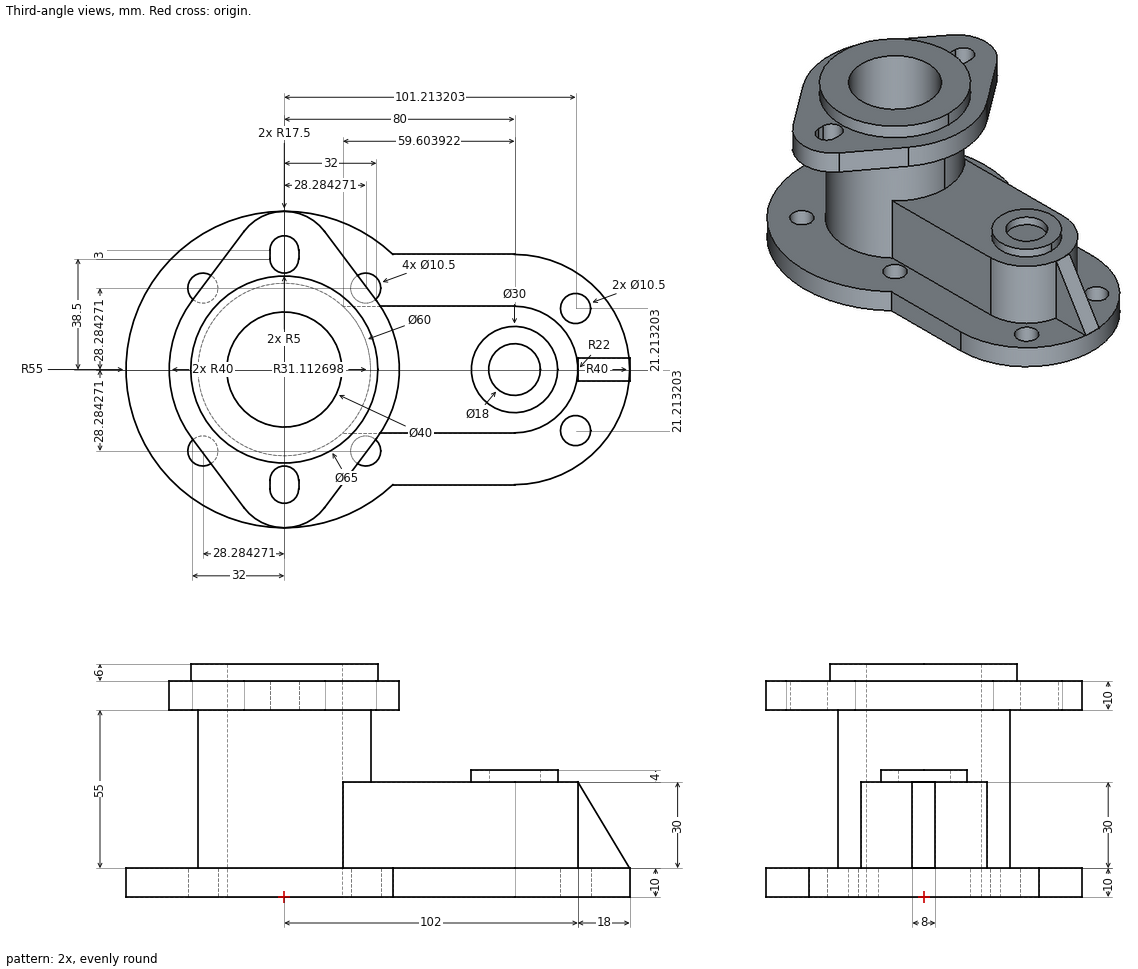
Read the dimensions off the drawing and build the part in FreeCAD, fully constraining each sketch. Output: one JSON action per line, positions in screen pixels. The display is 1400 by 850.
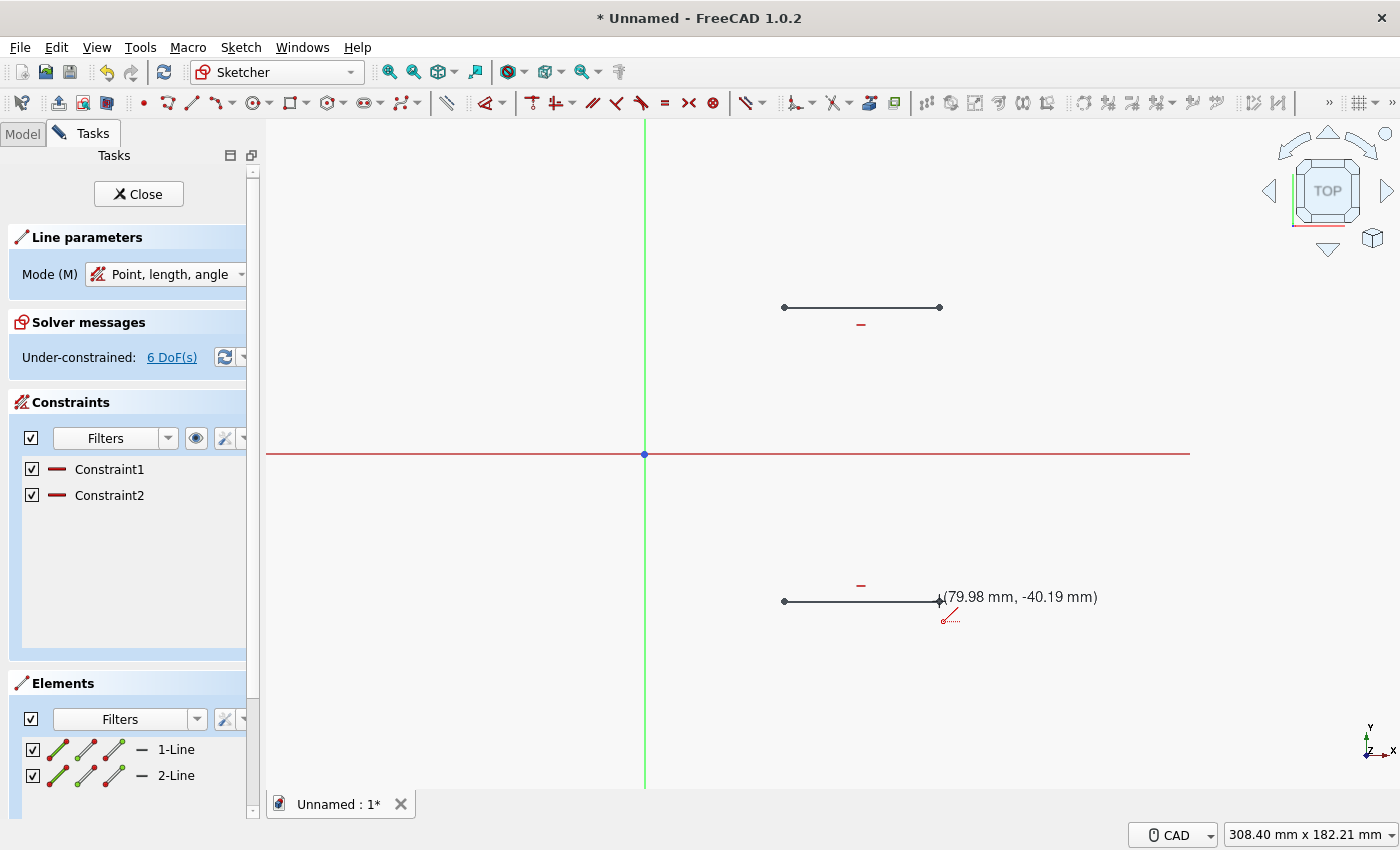
{"action": "key", "text": "g 3 a"}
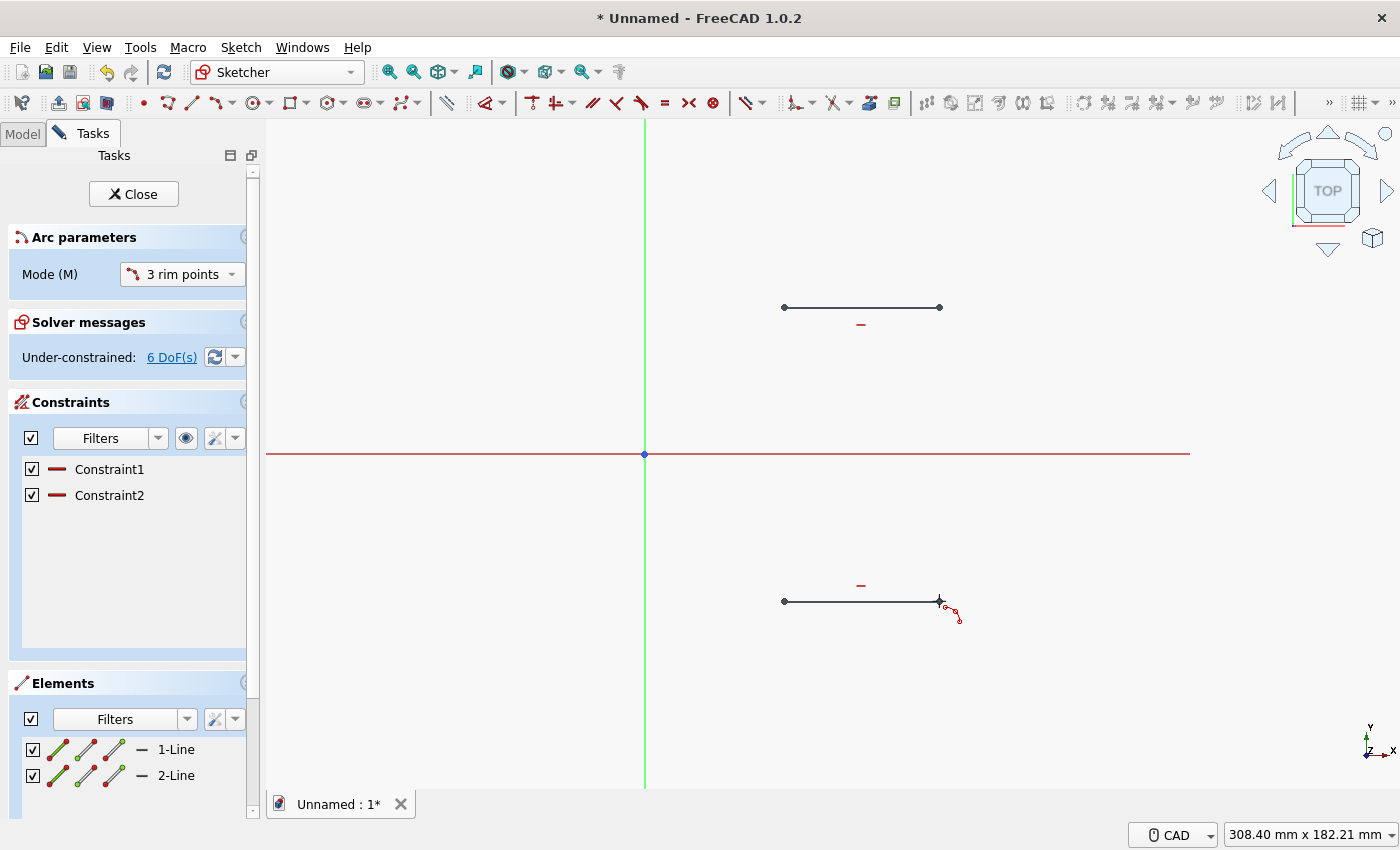
{"action": "left_click", "coordinate": [784, 308]}
{"action": "left_click", "coordinate": [784, 602]}
{"action": "left_click", "coordinate": [464, 363]}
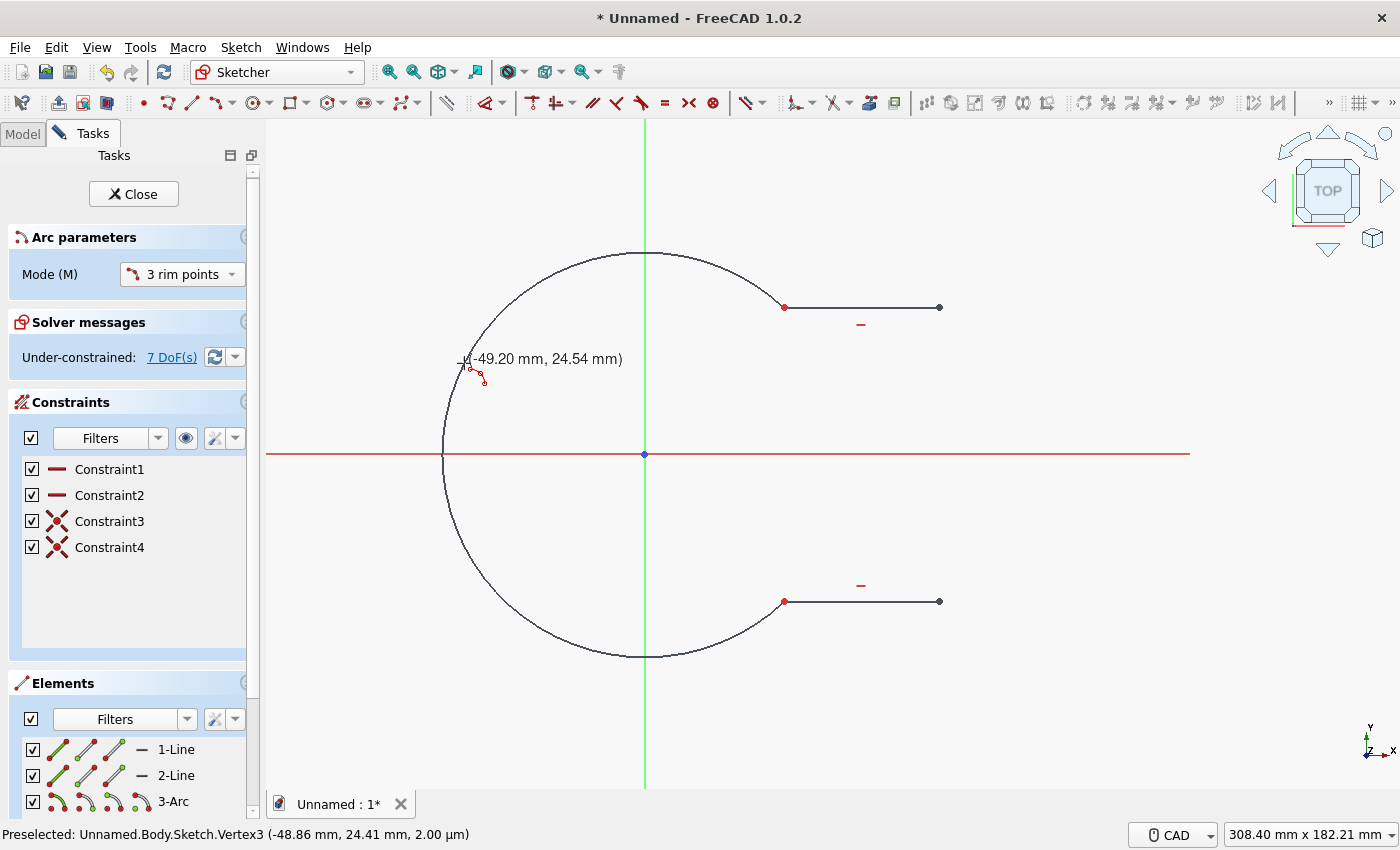
{"action": "left_click", "coordinate": [939, 602]}
{"action": "left_click", "coordinate": [939, 308]}
{"action": "left_click", "coordinate": [1079, 500]}
{"action": "key", "text": "Escape"}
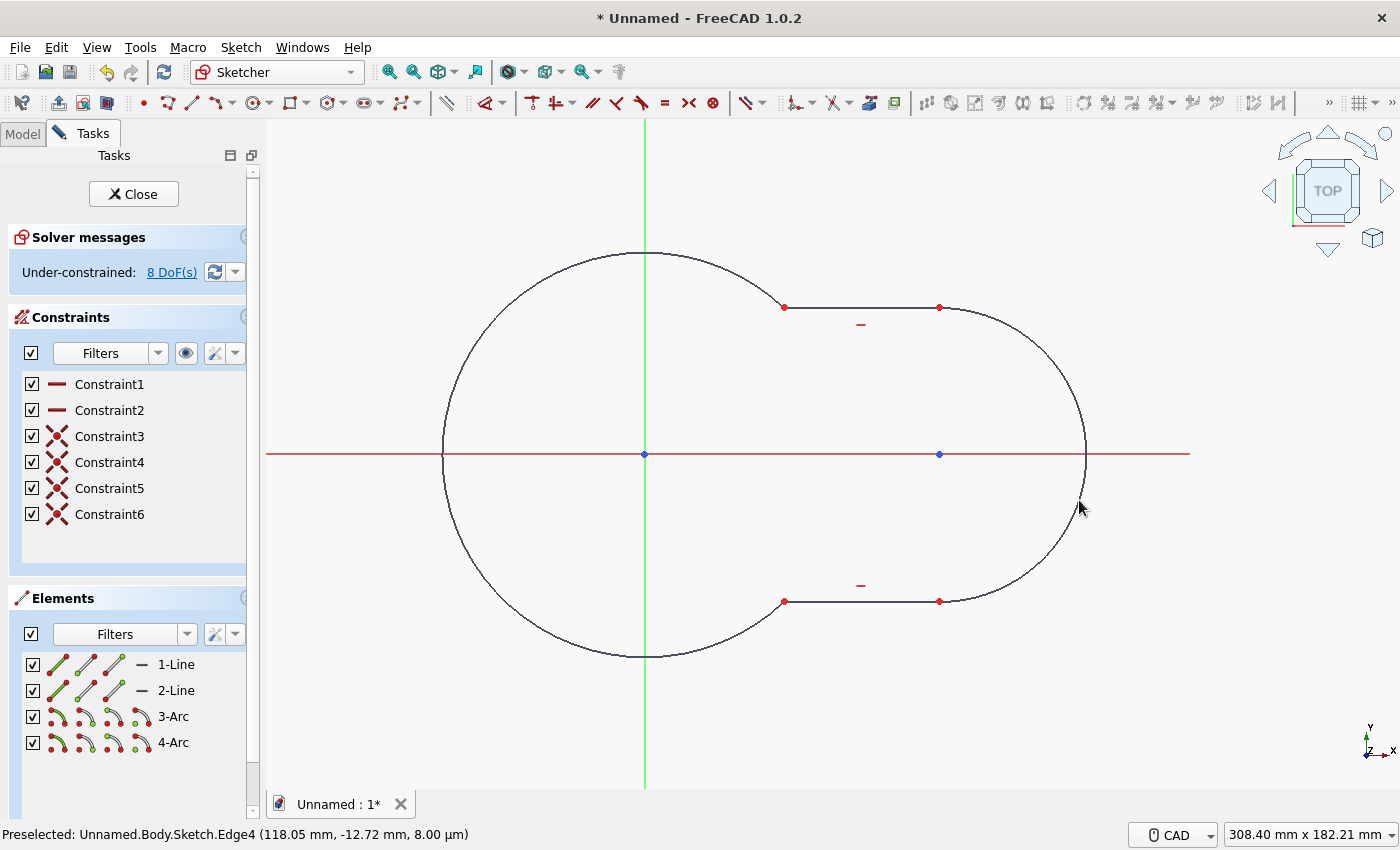
{"action": "left_click_drag", "start_coordinate": [635, 444], "coordinate": [655, 465]}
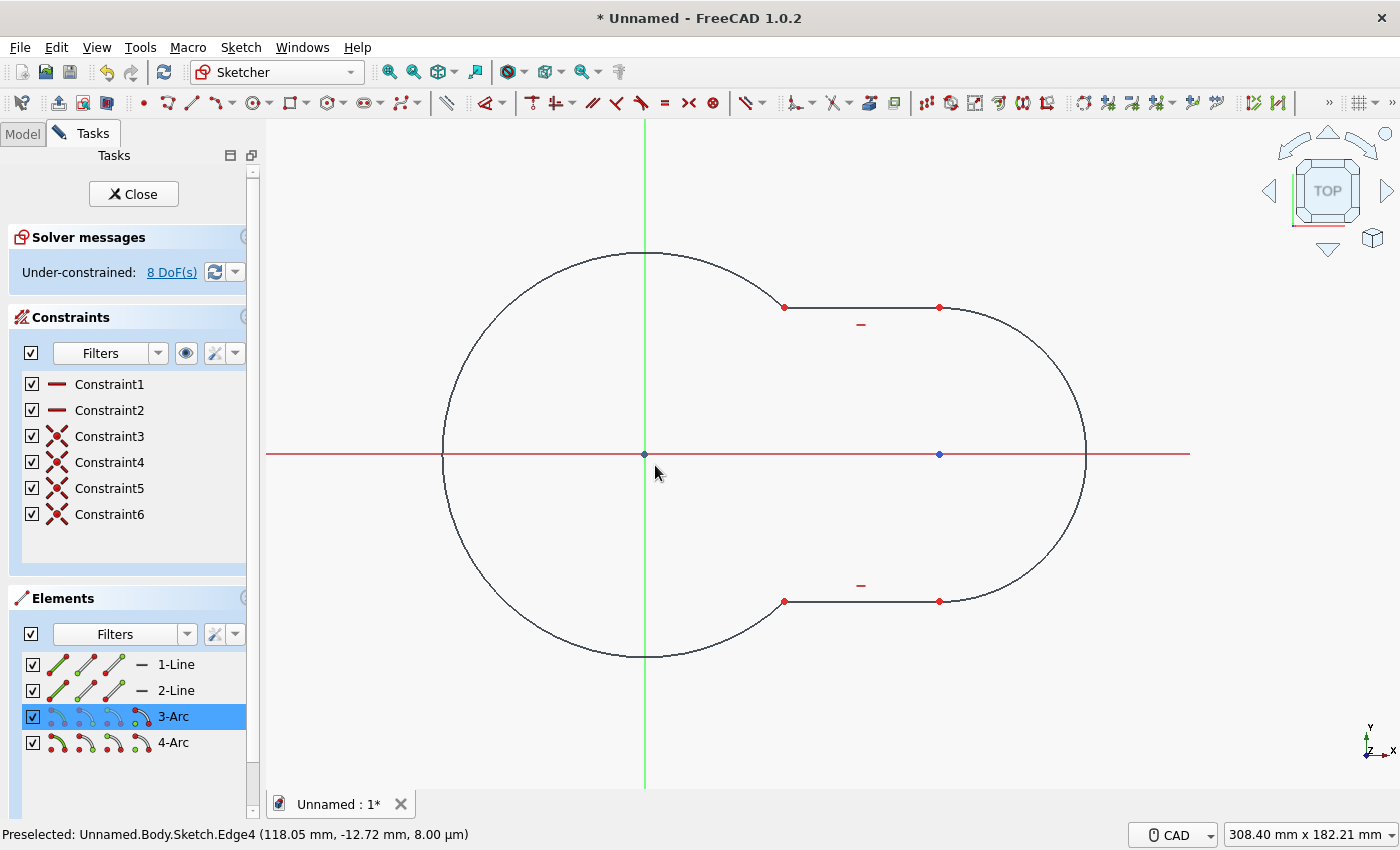
{"action": "key", "text": "c"}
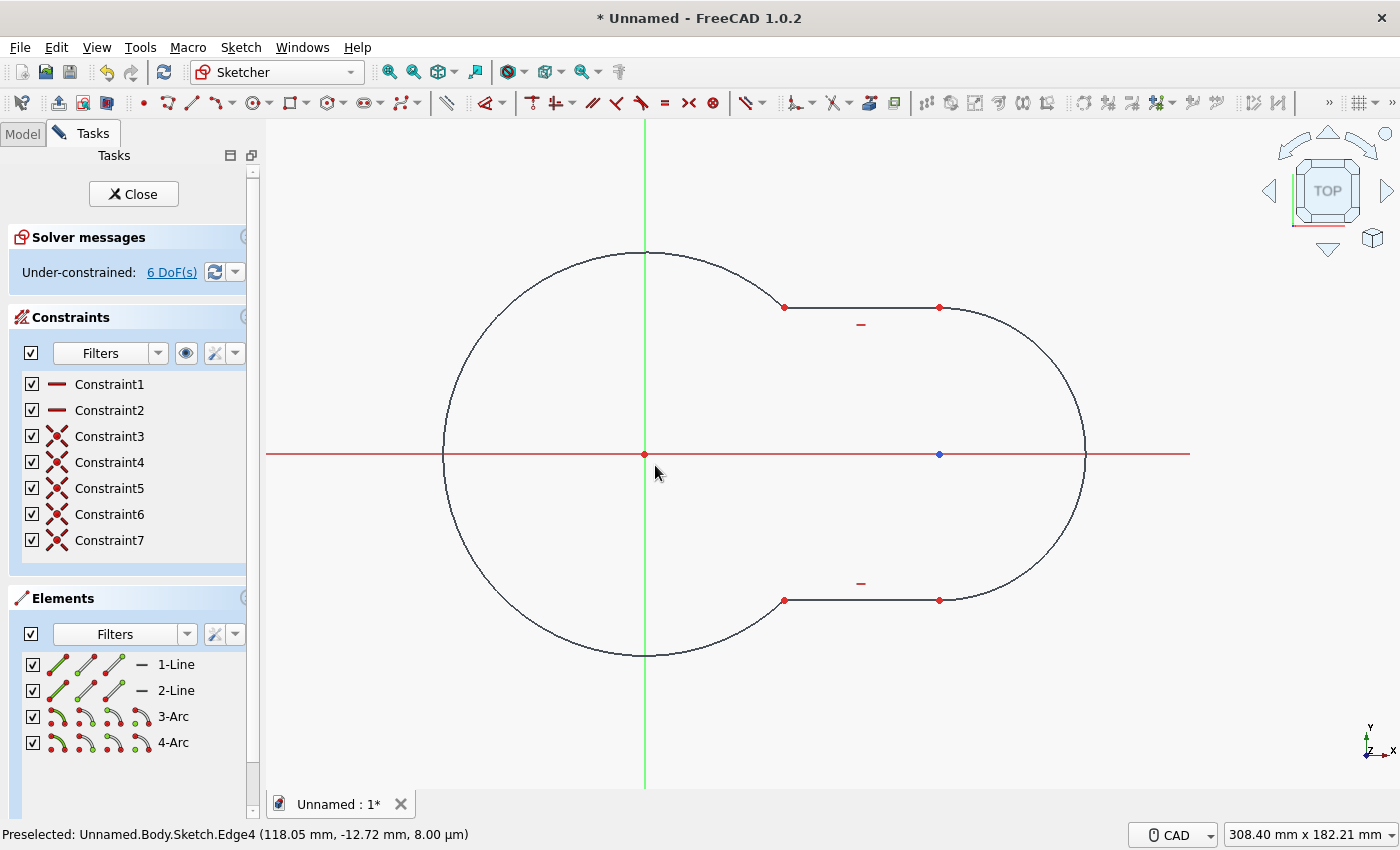
{"action": "left_click", "coordinate": [939, 454]}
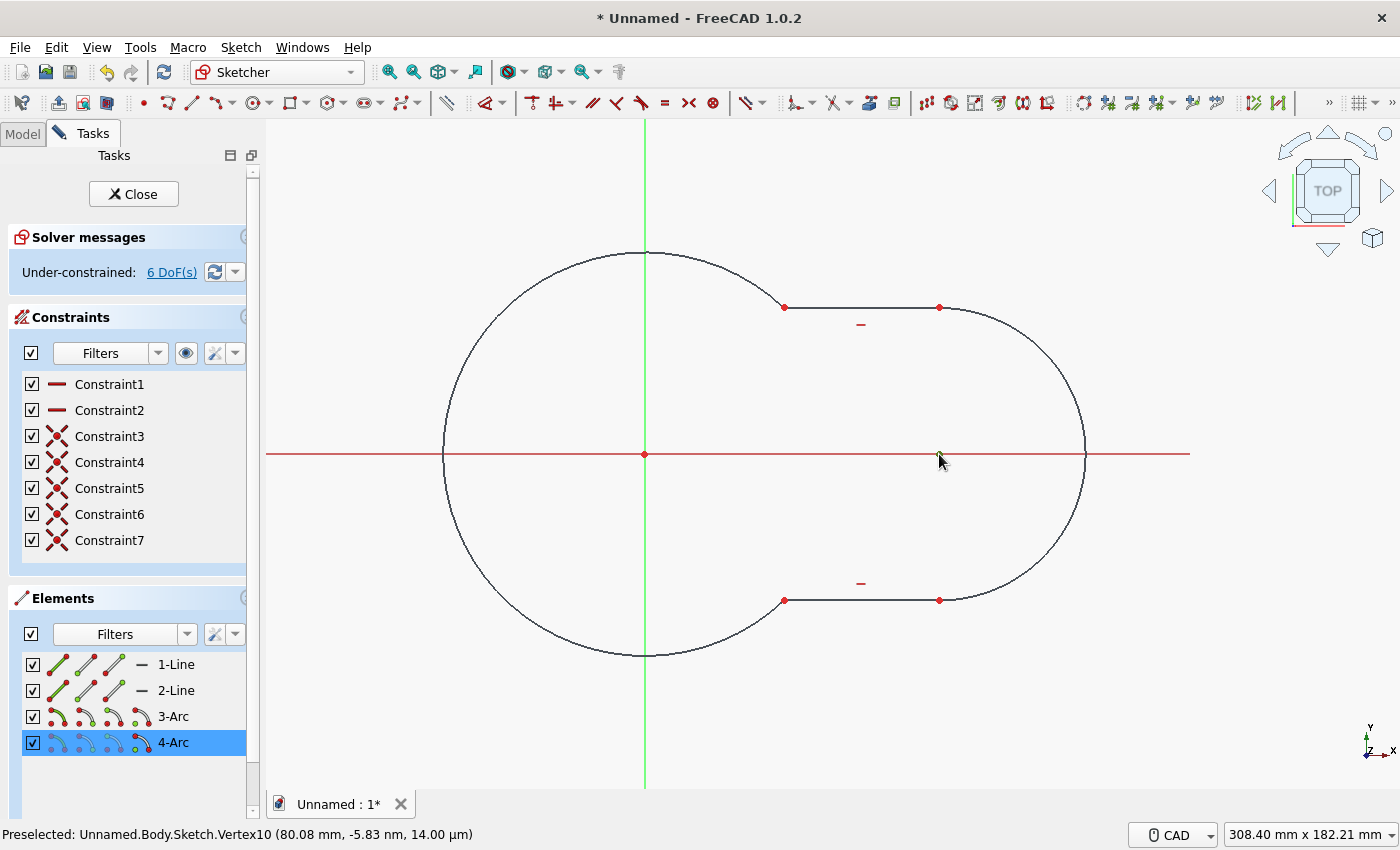
{"action": "left_click", "coordinate": [361, 454]}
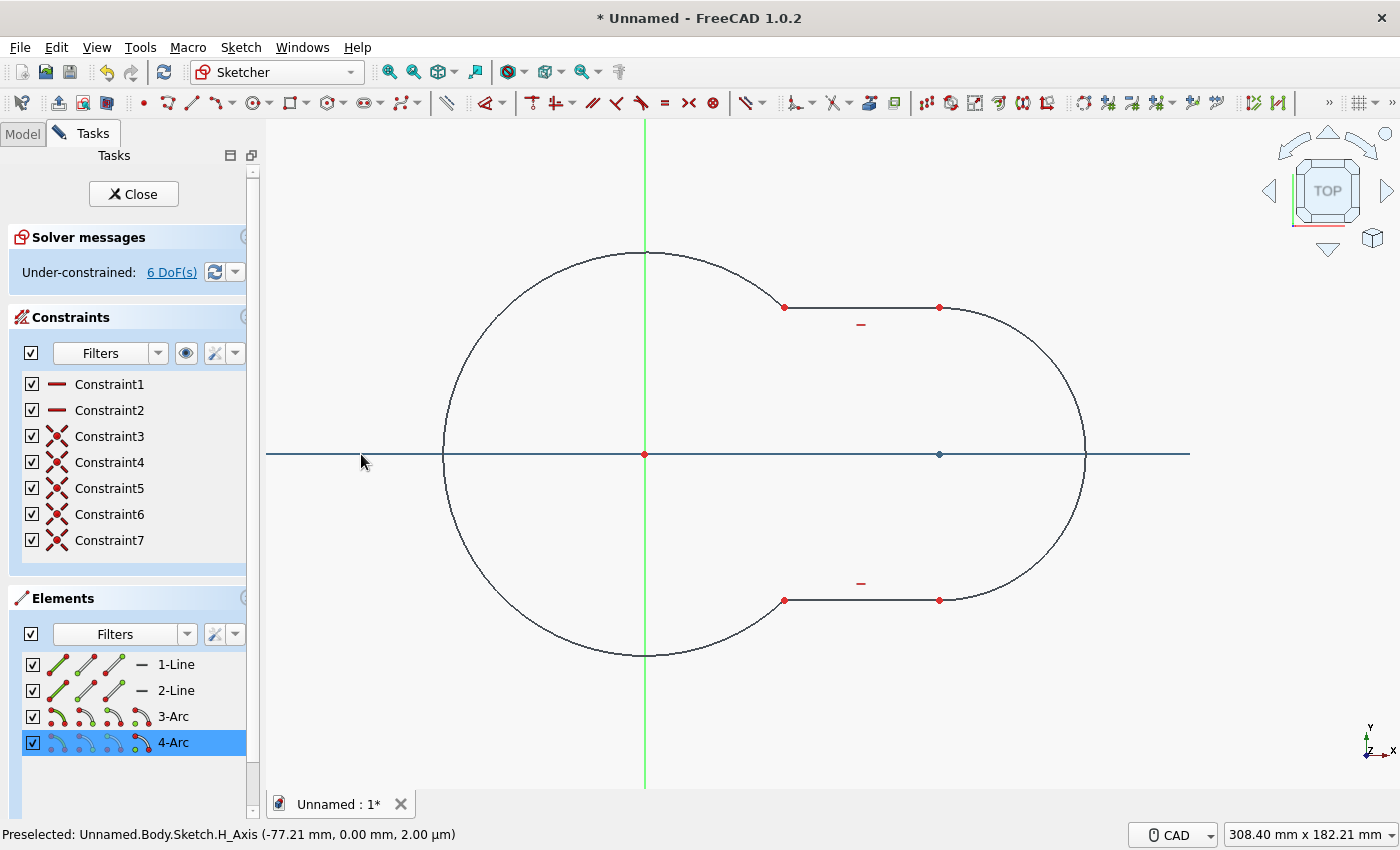
{"action": "key", "text": "c"}